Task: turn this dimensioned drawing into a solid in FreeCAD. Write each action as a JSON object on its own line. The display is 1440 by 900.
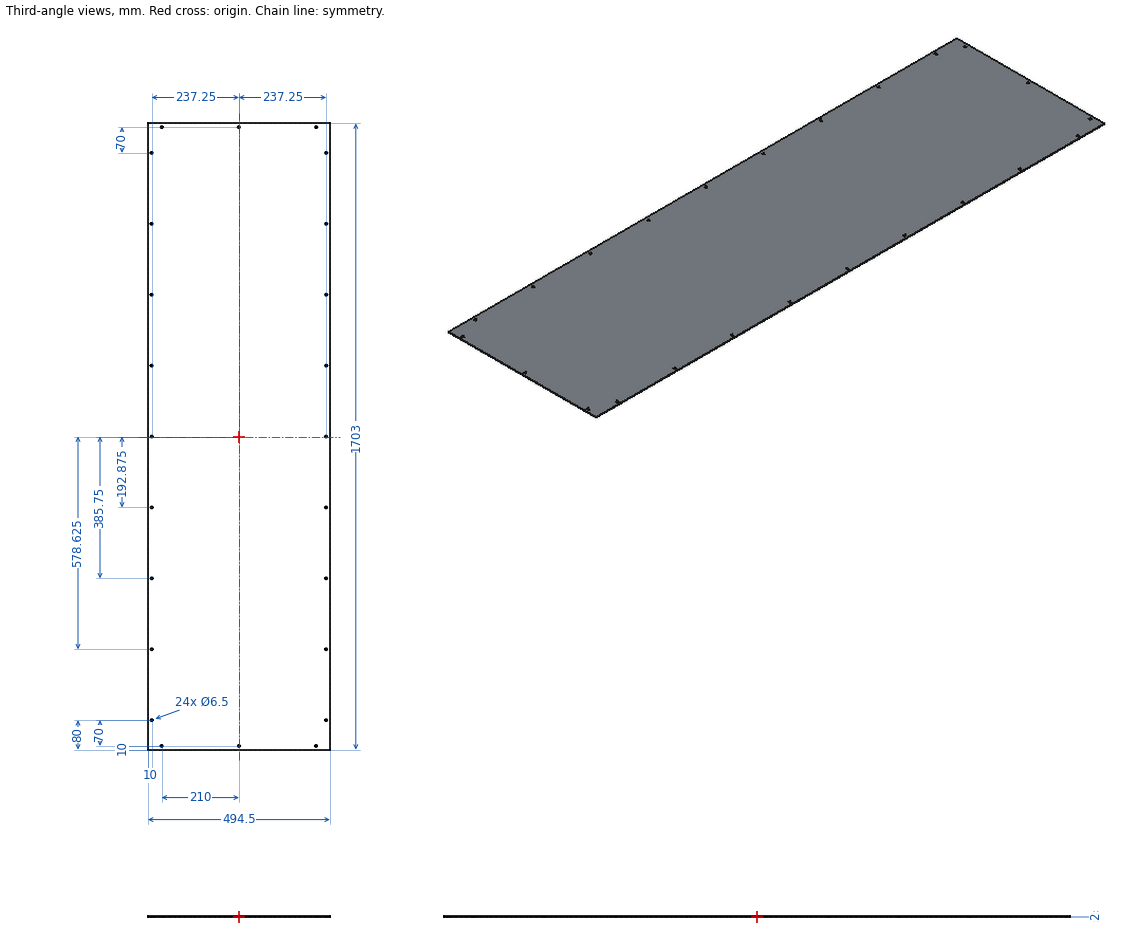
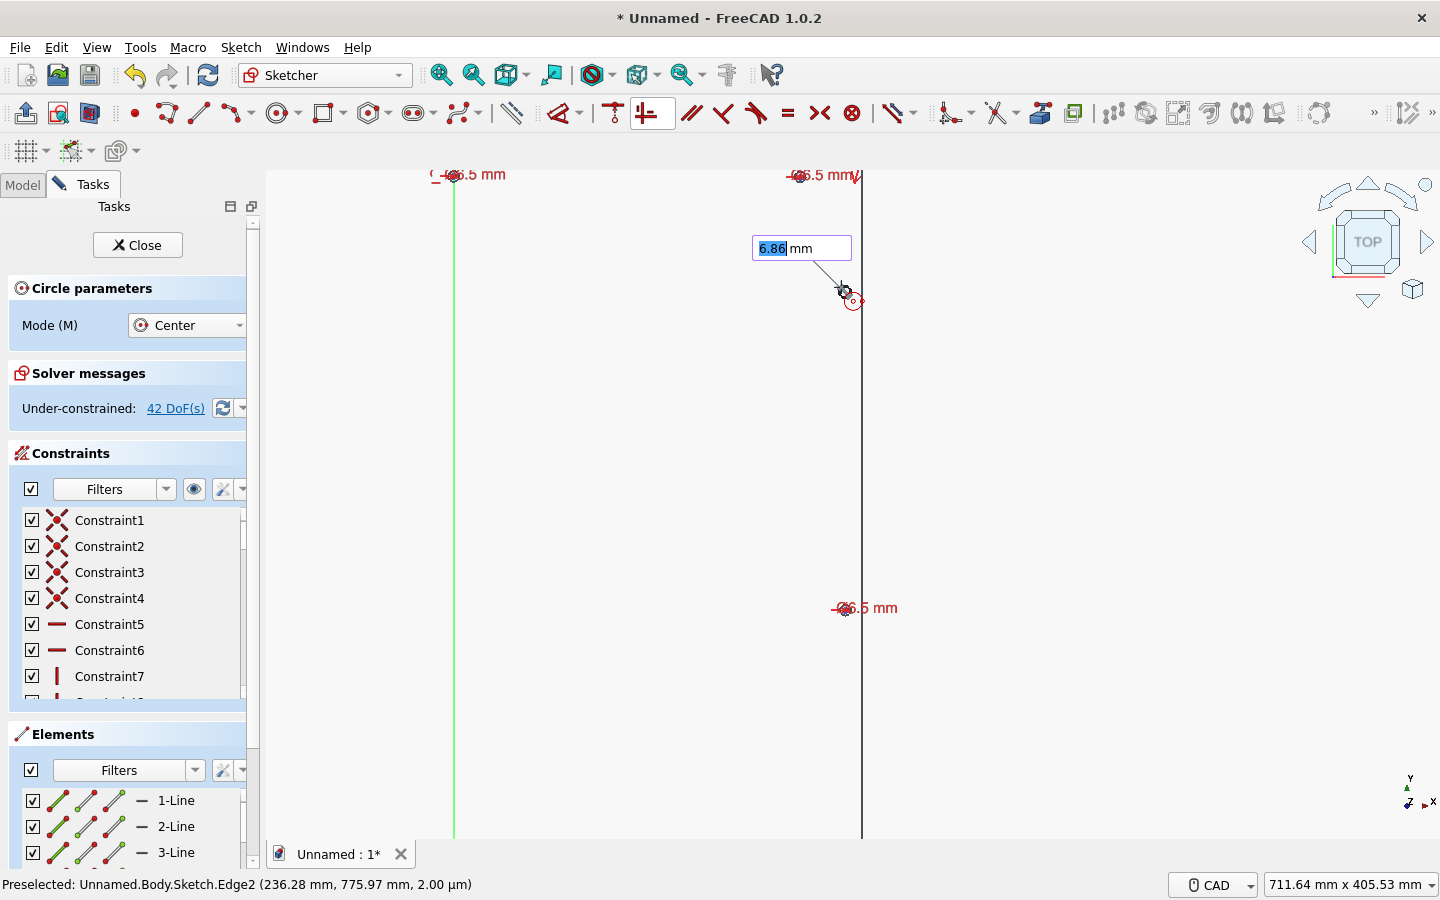
{"action": "type", "text": "6.5"}
{"action": "key", "text": "Return"}
{"action": "key", "text": "Escape"}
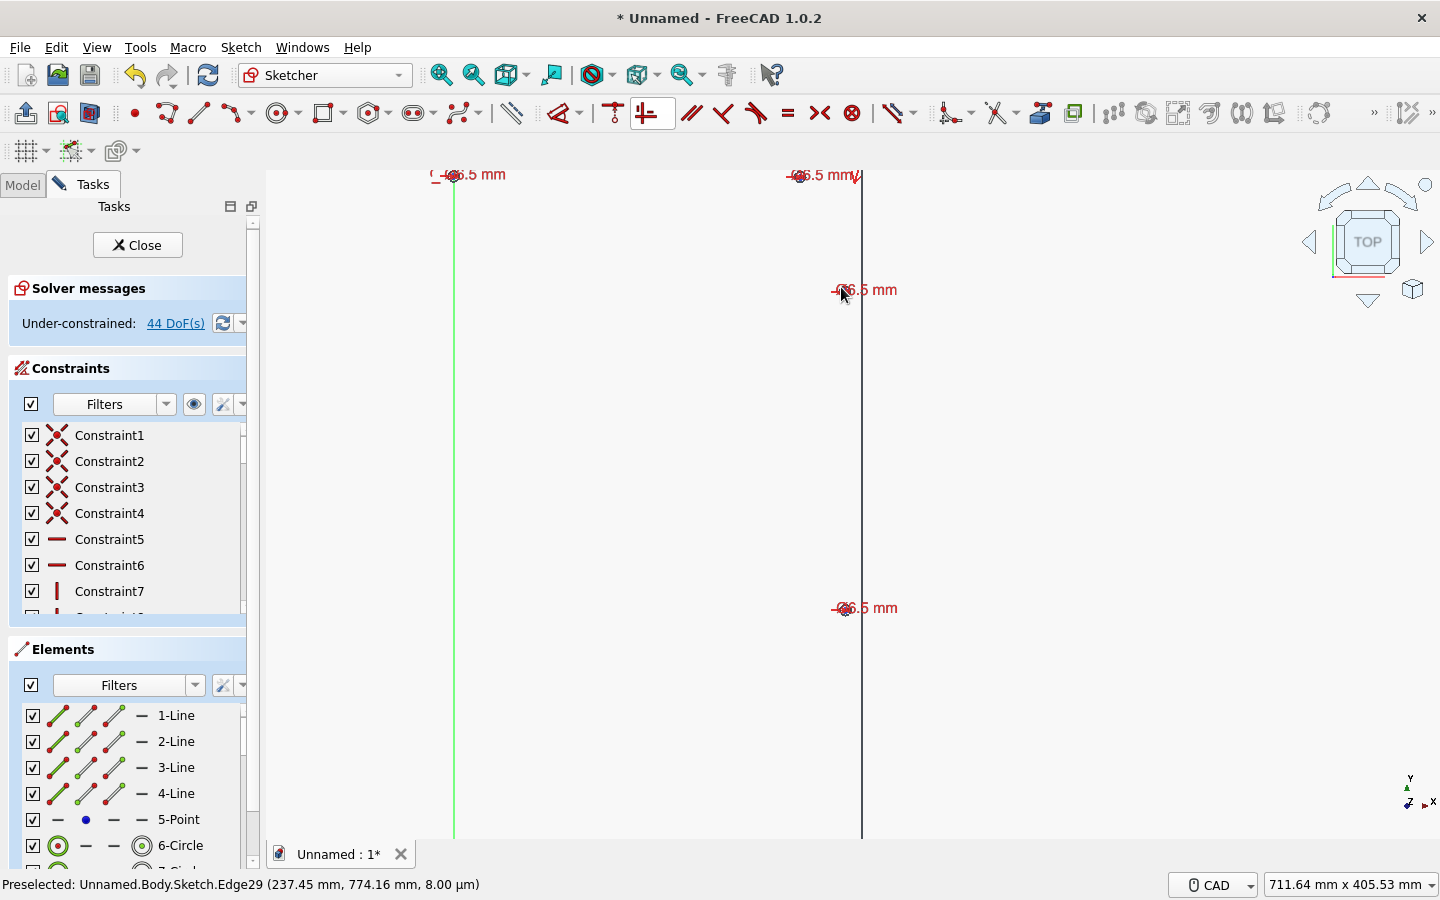
{"action": "scroll", "coordinate": [850, 295], "scroll_direction": "down", "scroll_amount": 9}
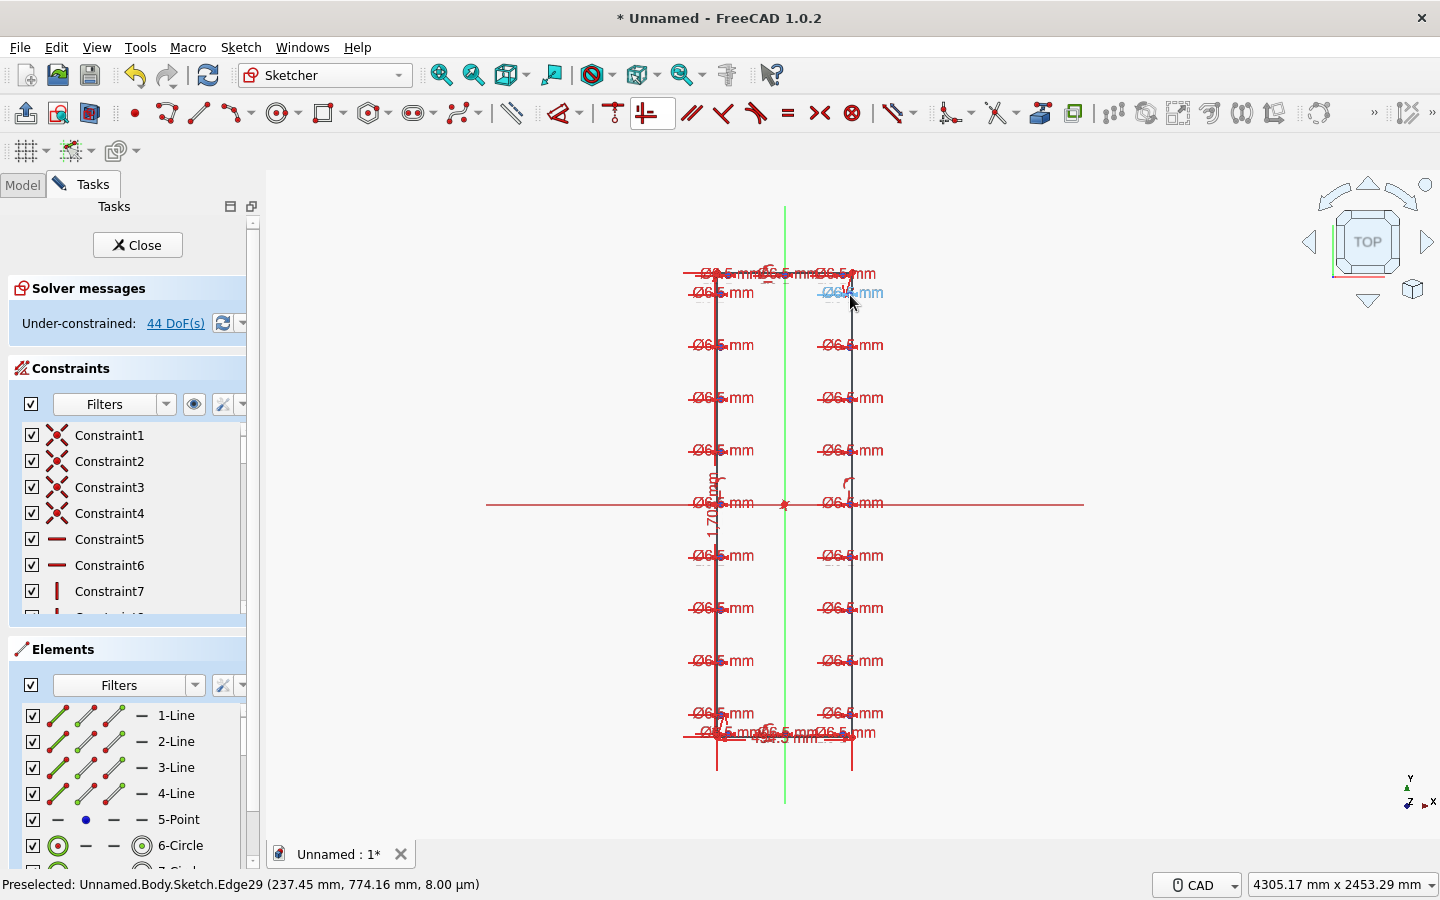
{"action": "left_click", "coordinate": [728, 734]}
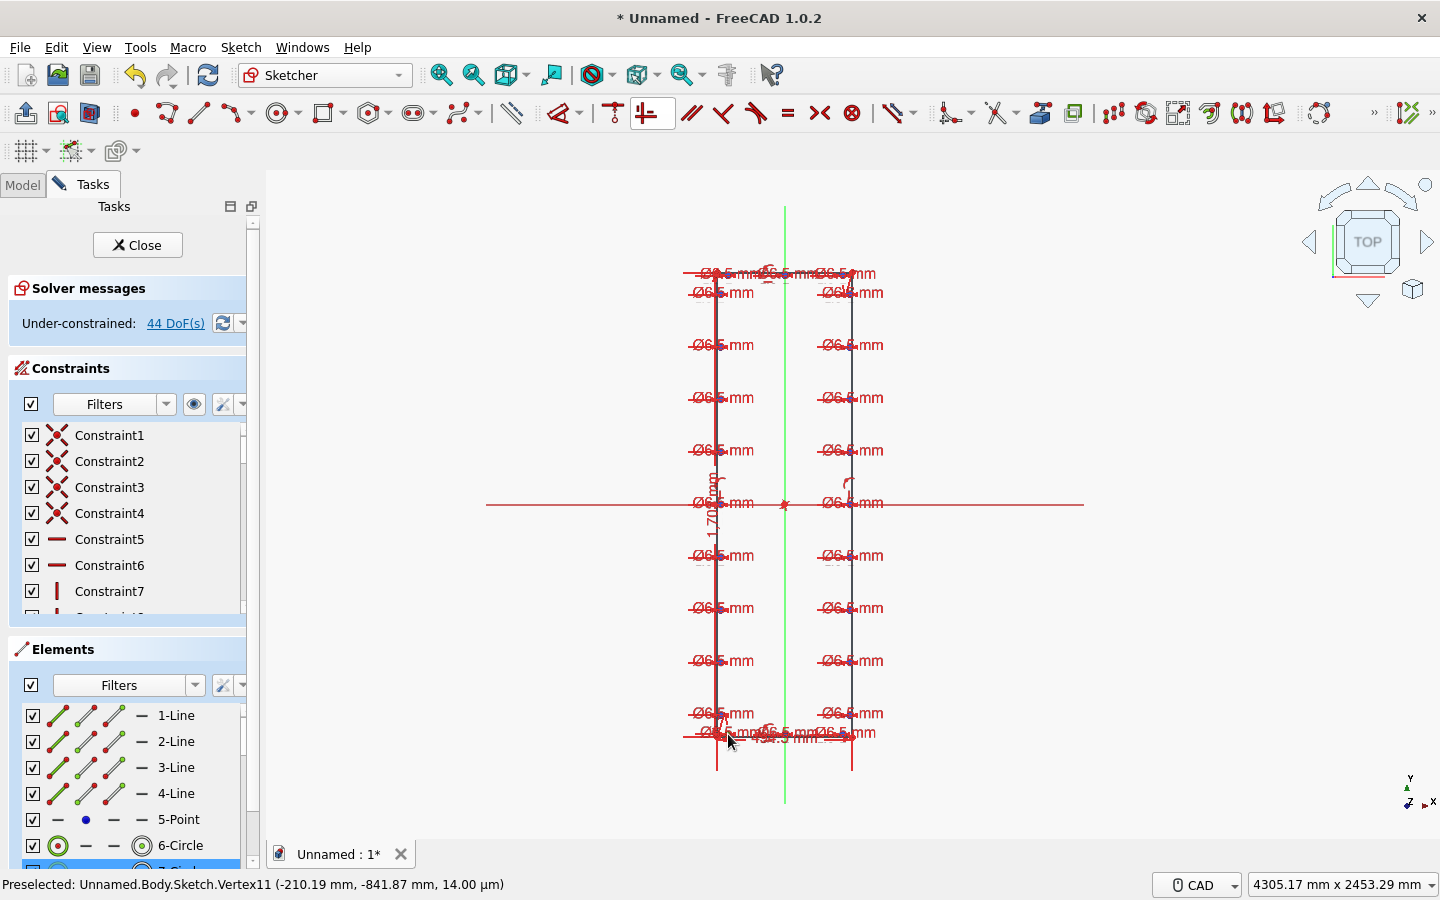
{"action": "left_click", "coordinate": [842, 735]}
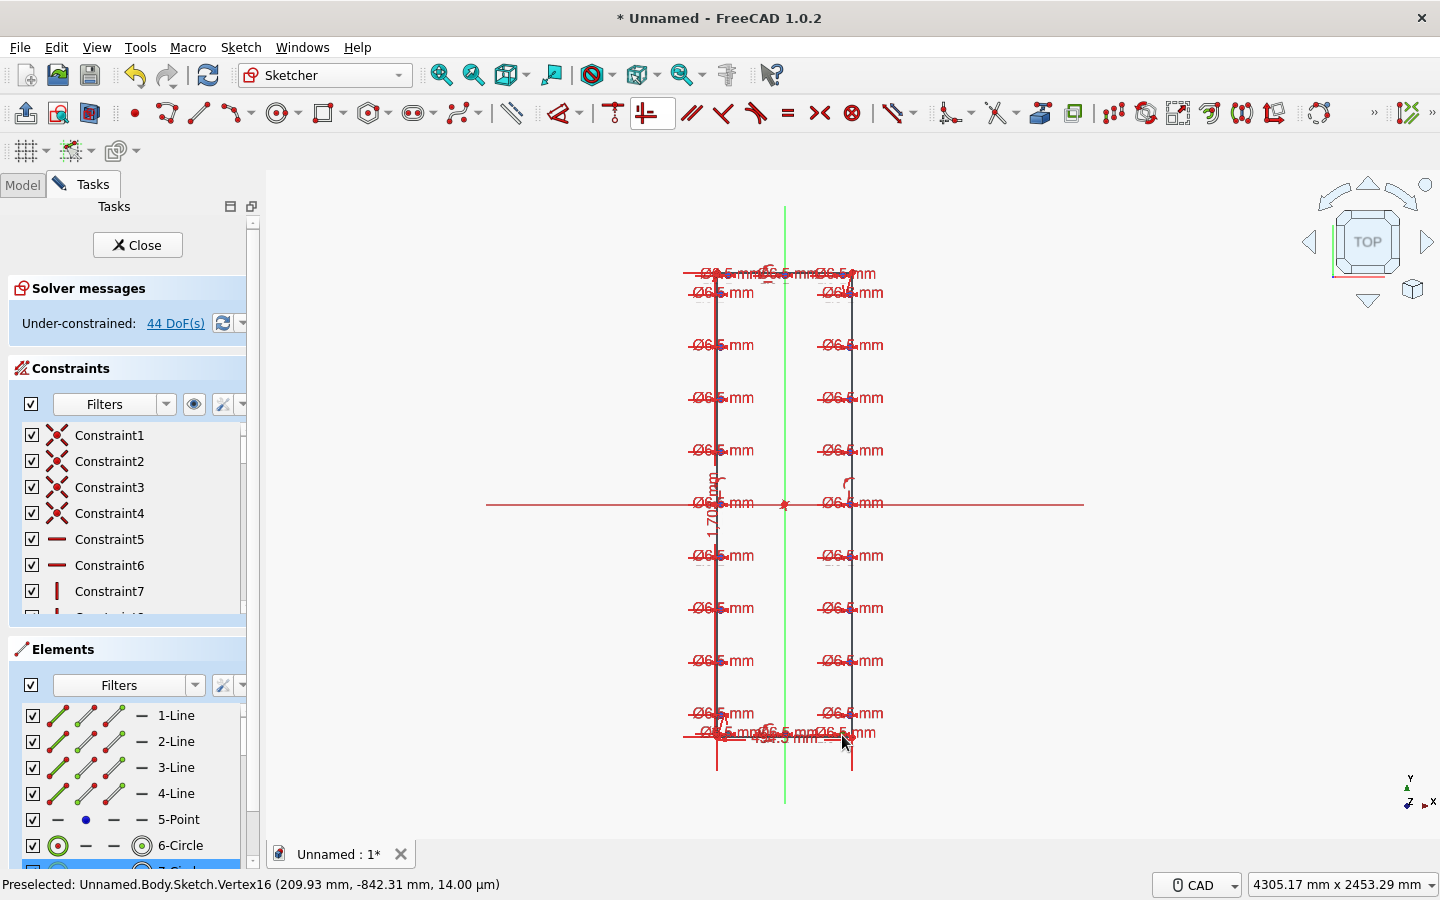
{"action": "left_click", "coordinate": [785, 767]}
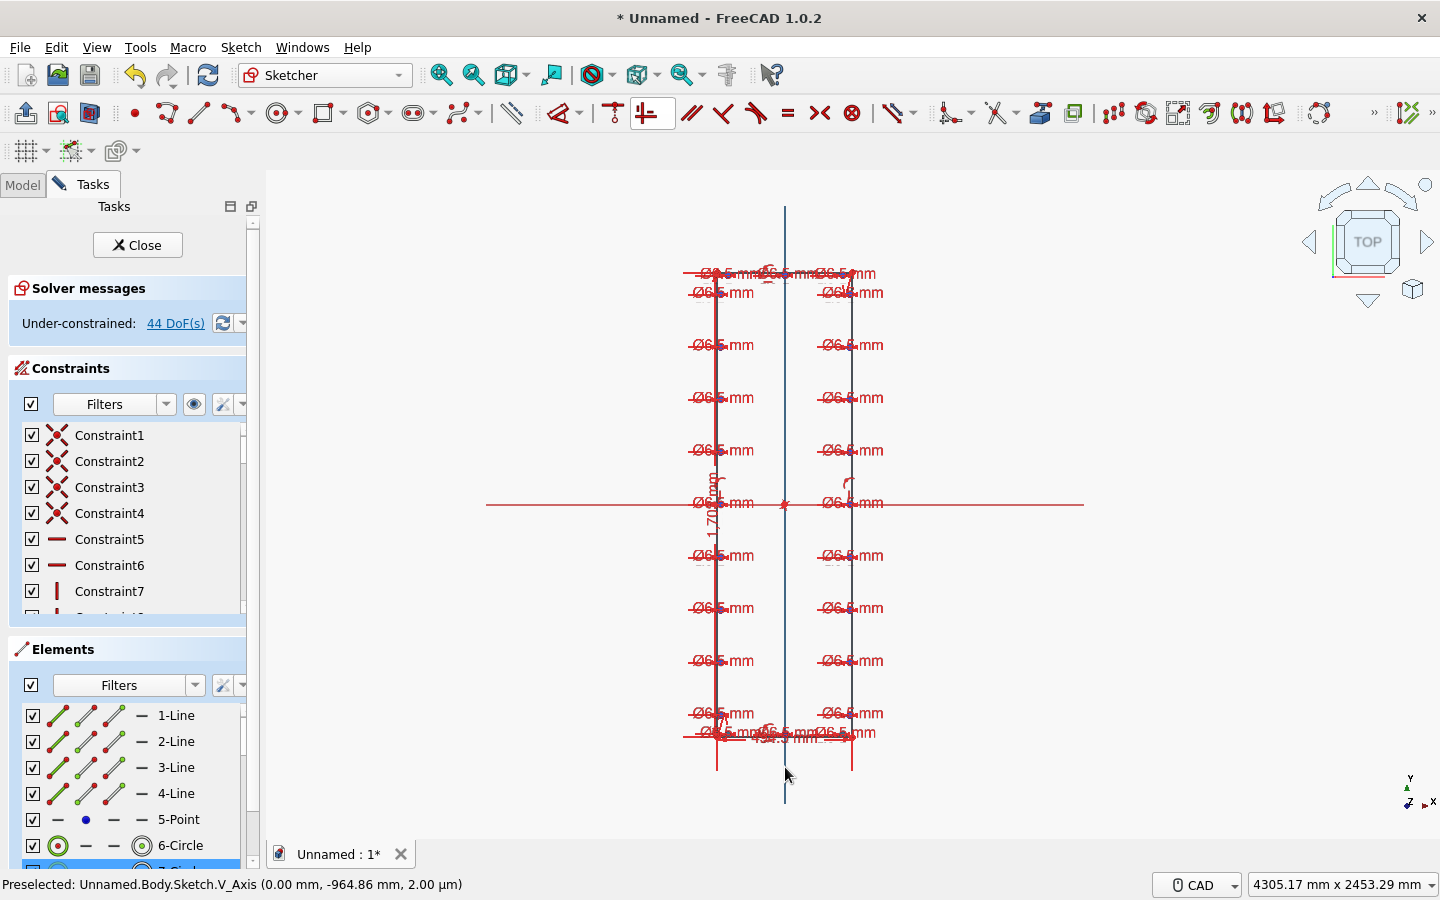
{"action": "left_click", "coordinate": [820, 114]}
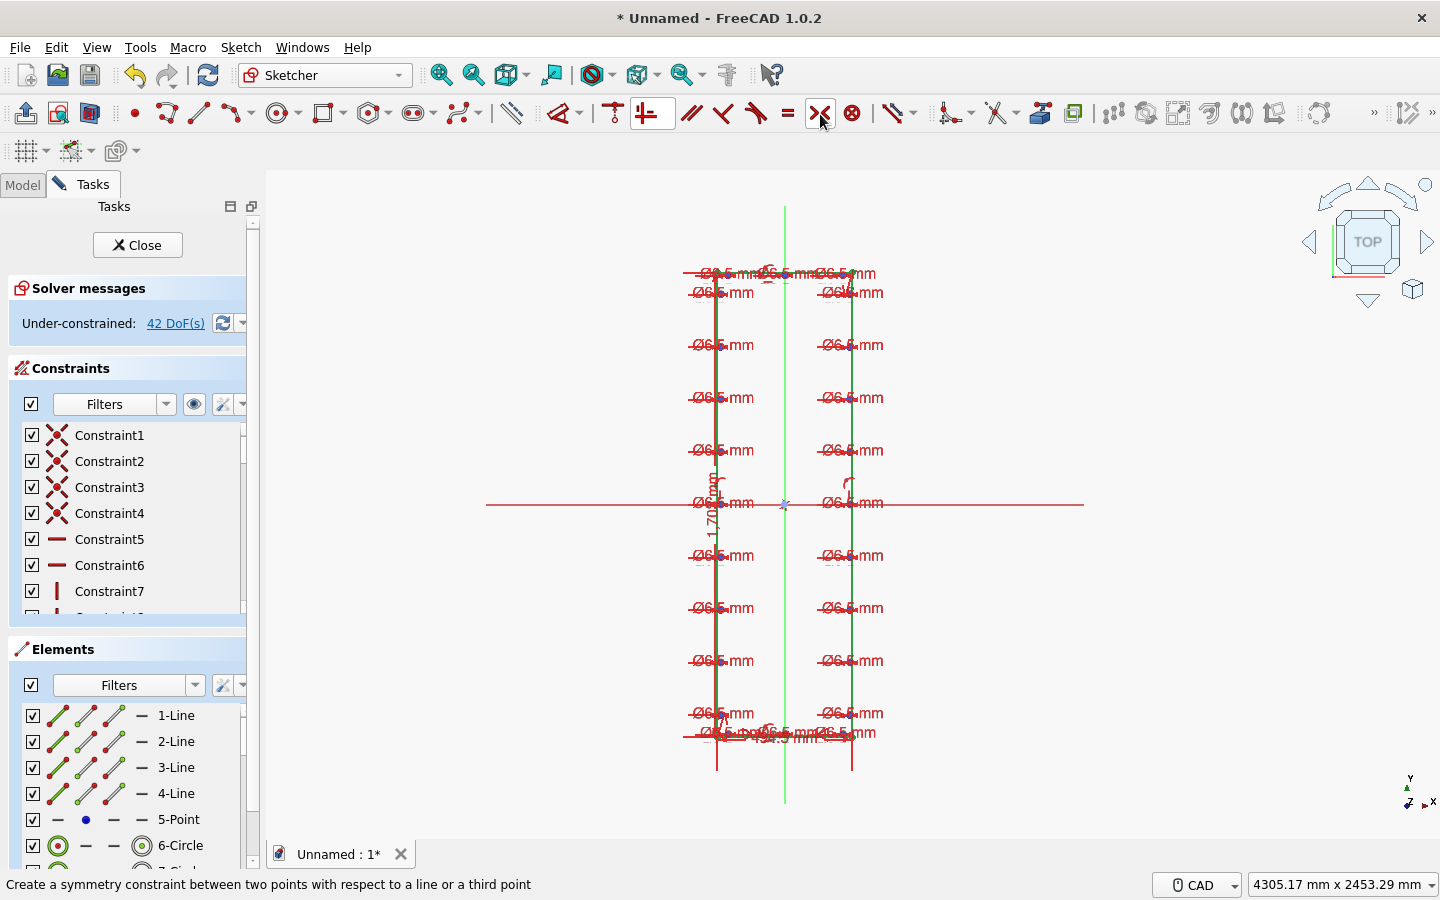
{"action": "left_click", "coordinate": [720, 715]}